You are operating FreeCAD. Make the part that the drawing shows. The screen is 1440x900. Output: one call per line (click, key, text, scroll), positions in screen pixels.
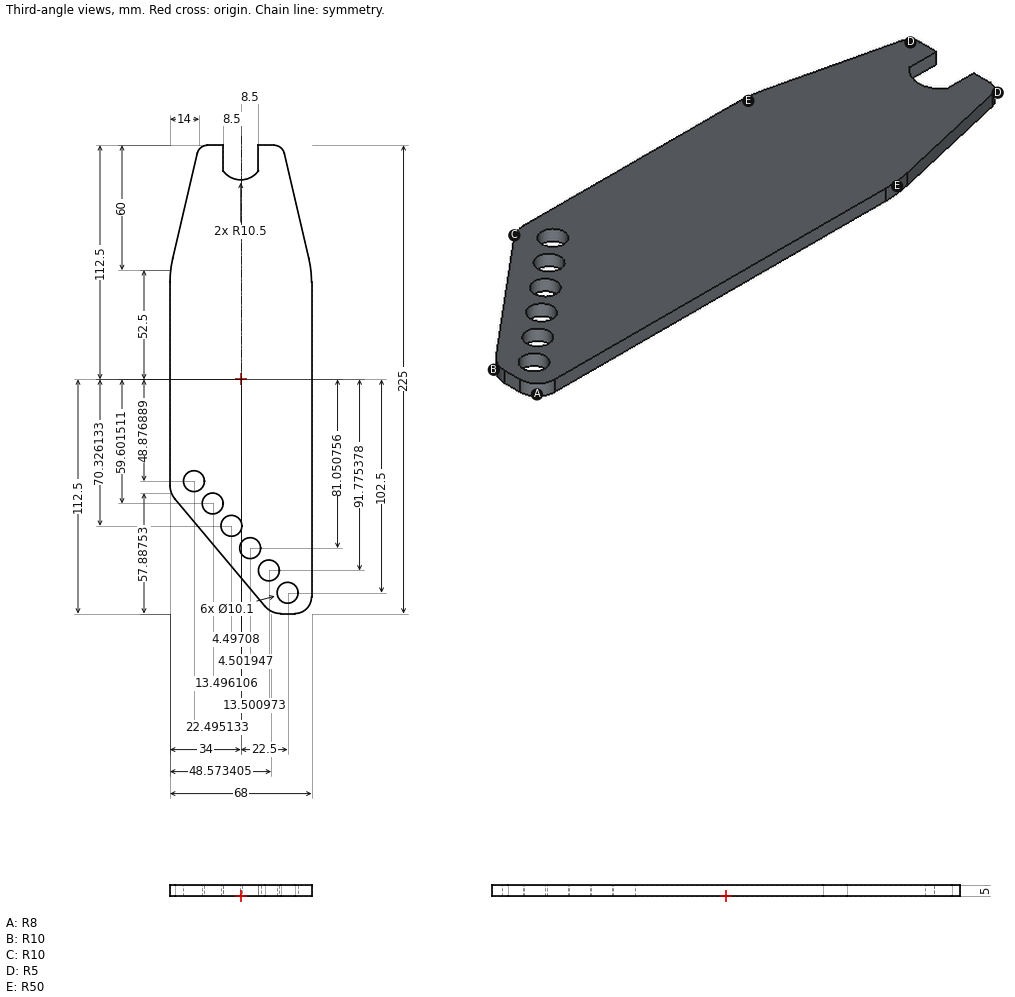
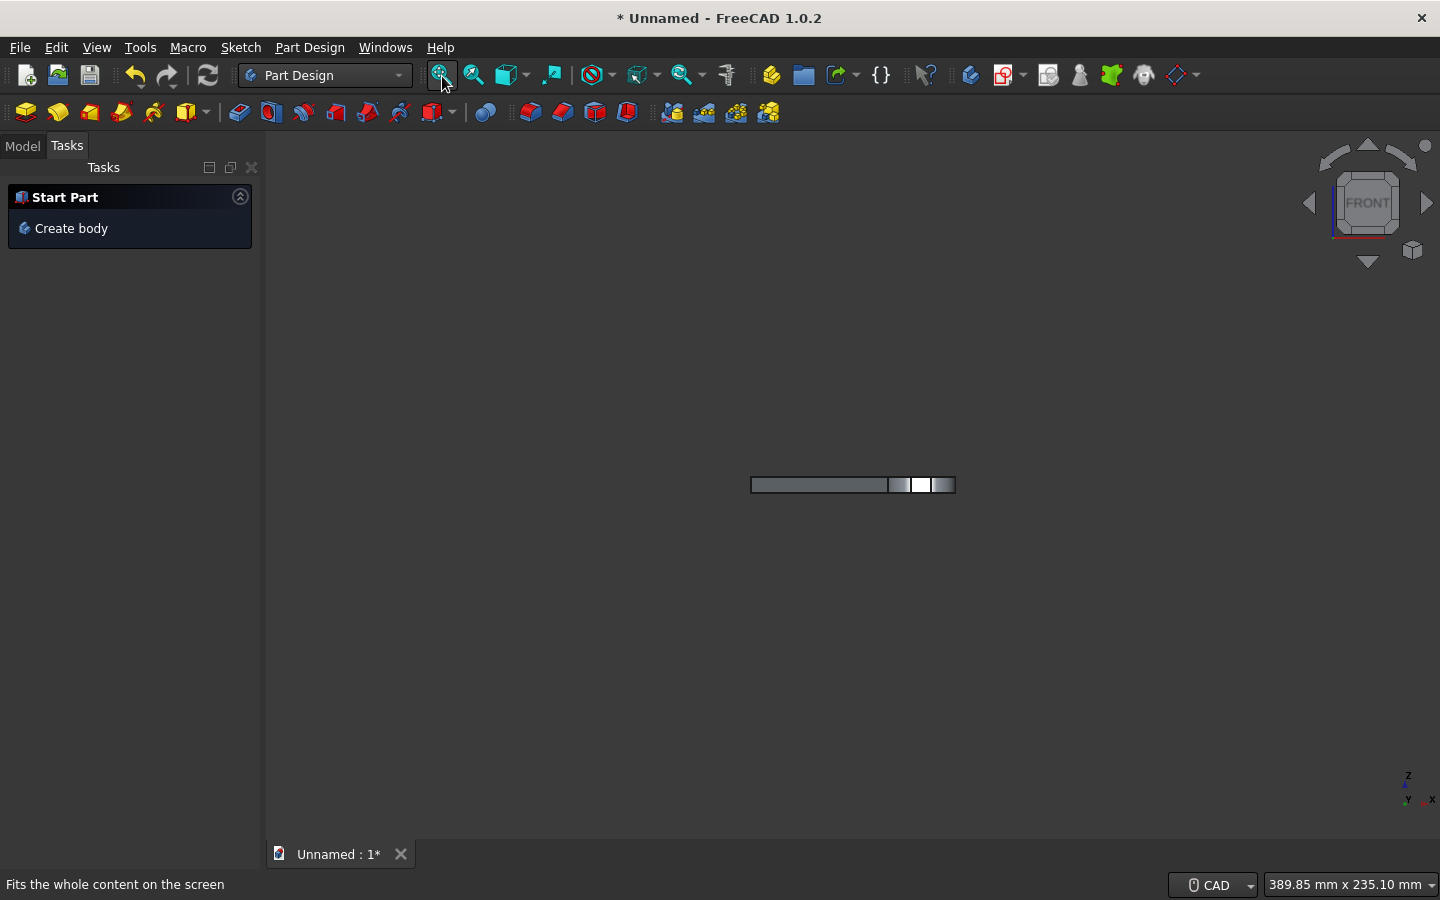
key(0)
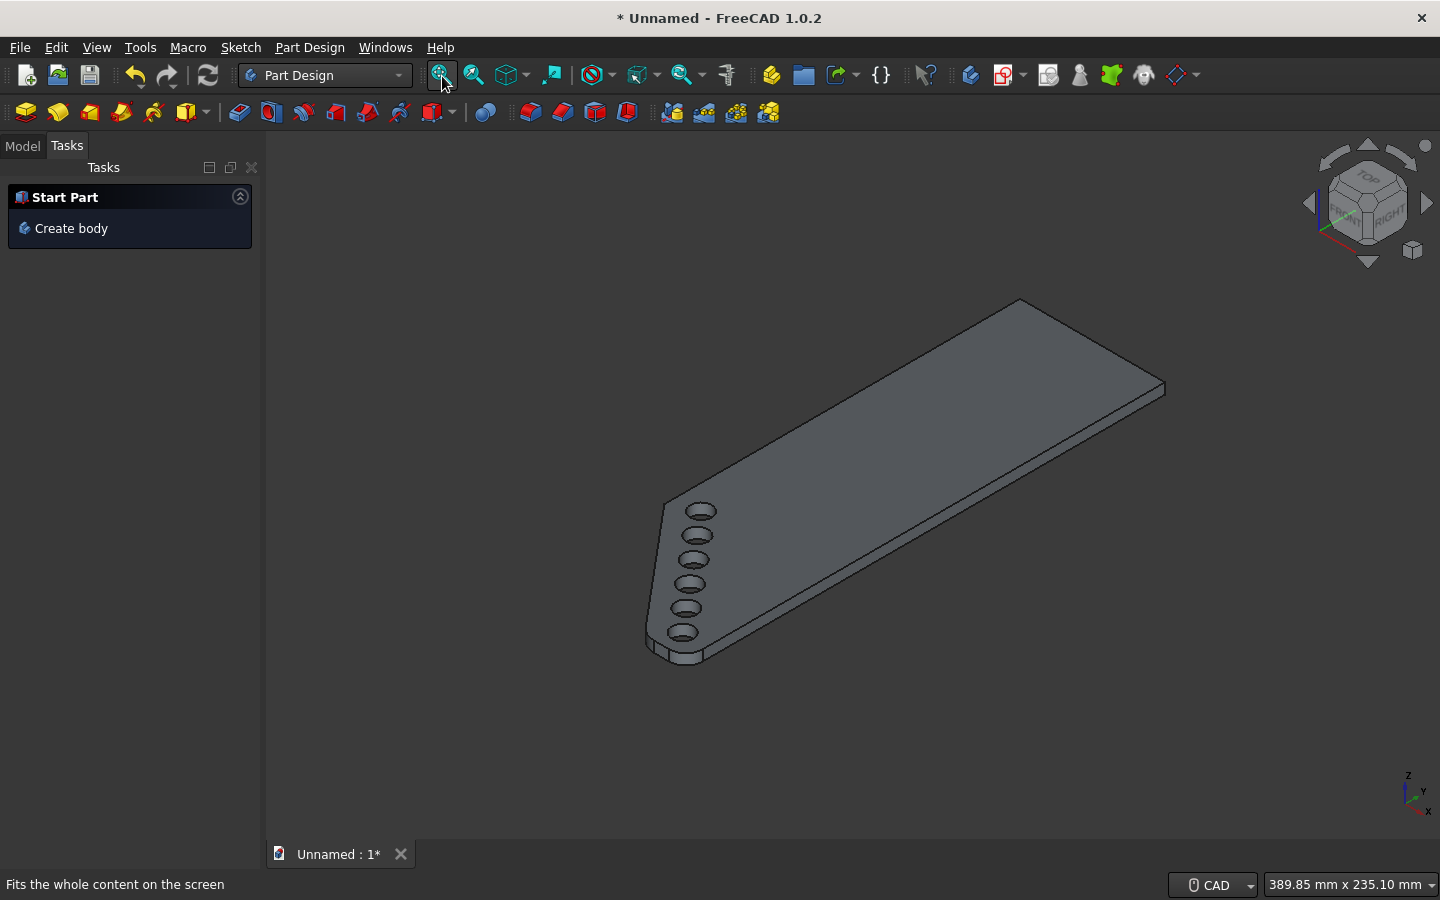
click(990, 399)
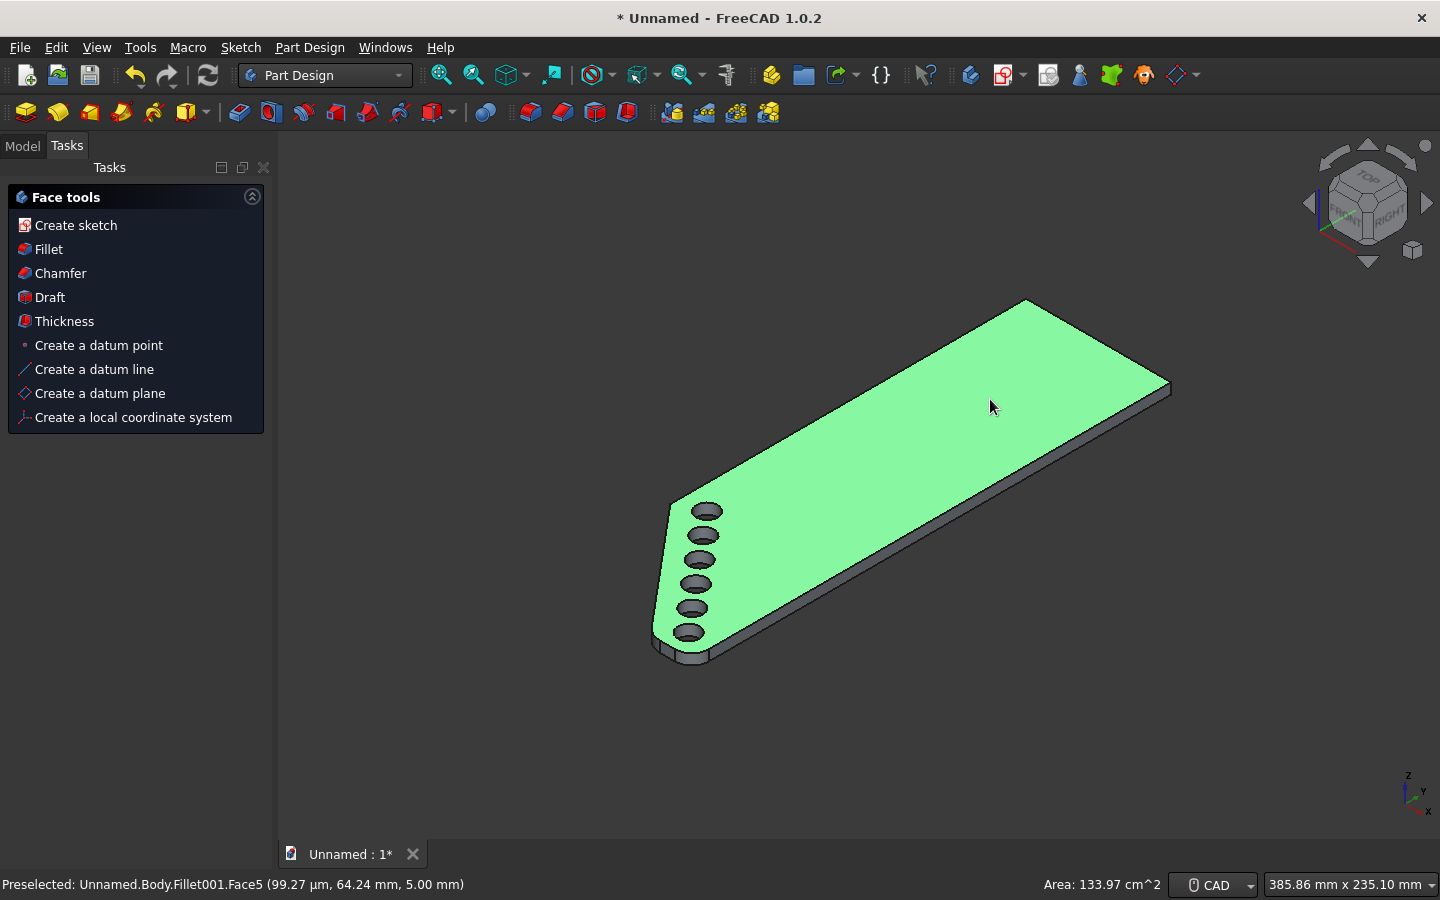
click(1004, 76)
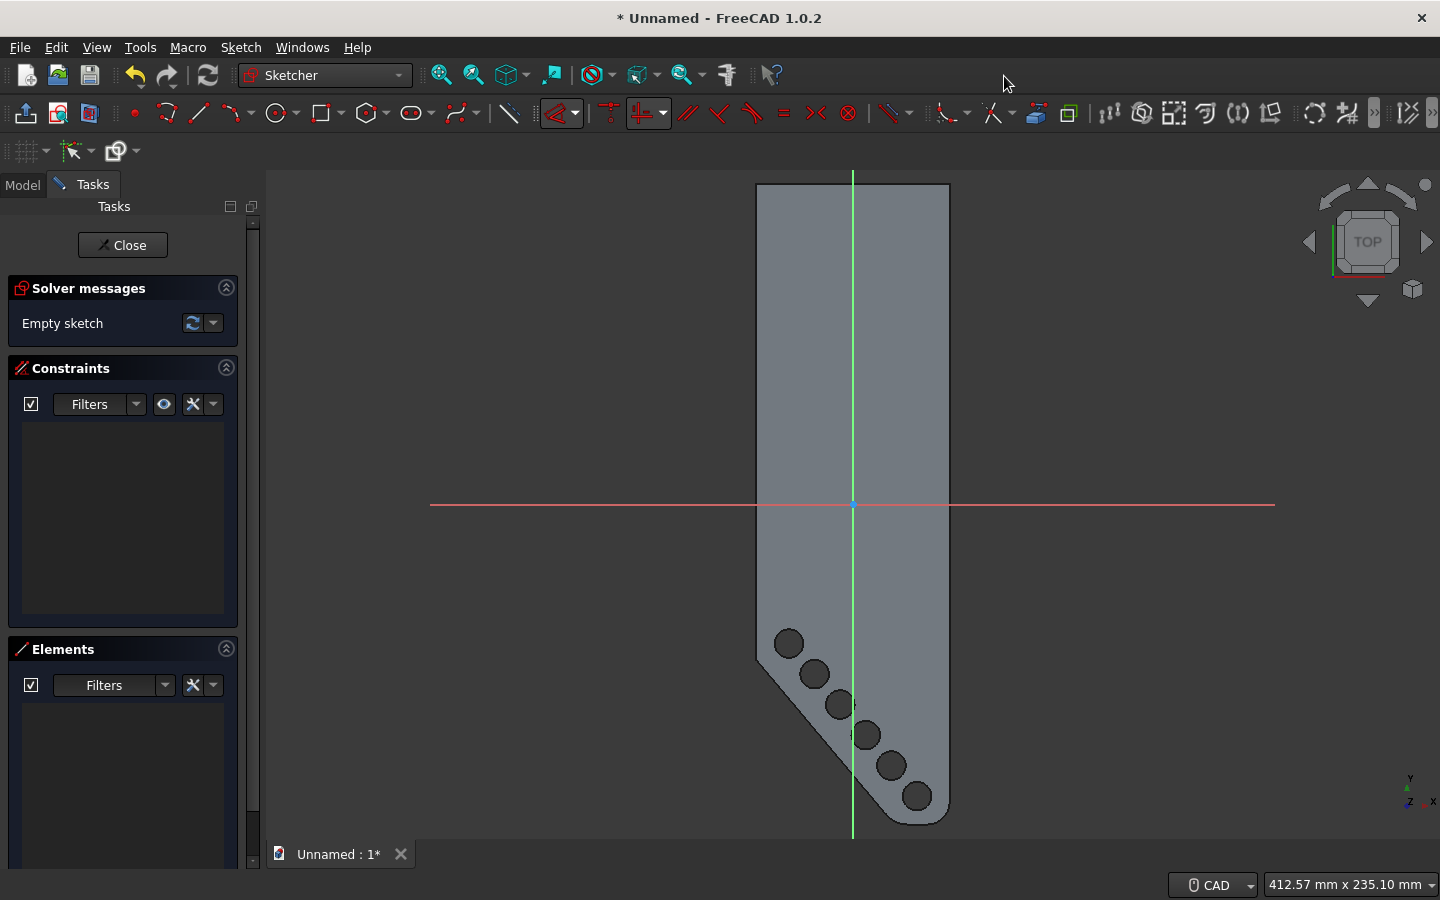
scroll(784, 504, down, 5)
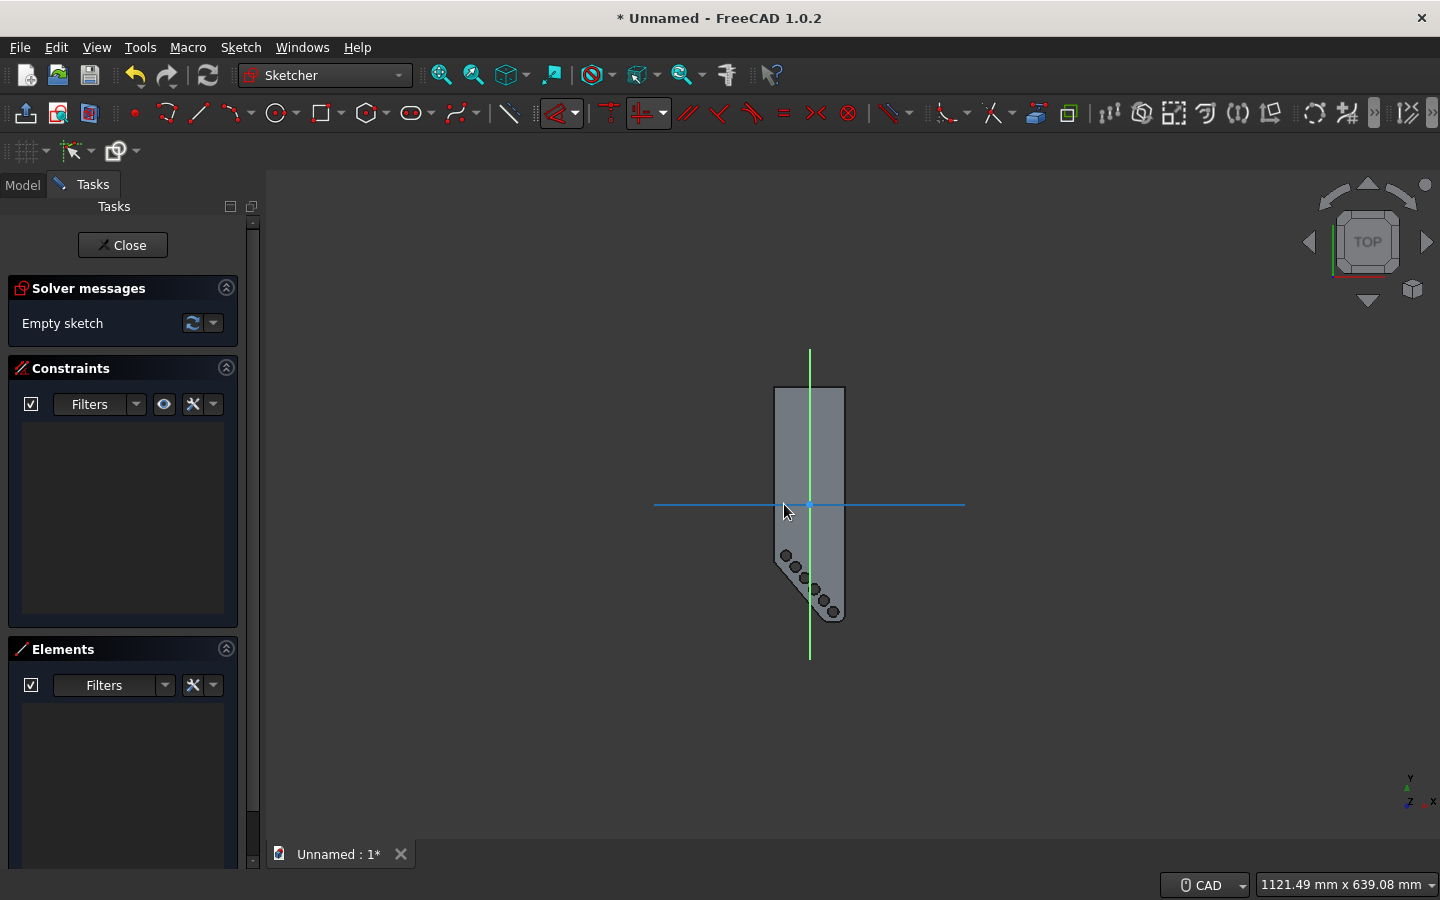
scroll(811, 387, up, 15)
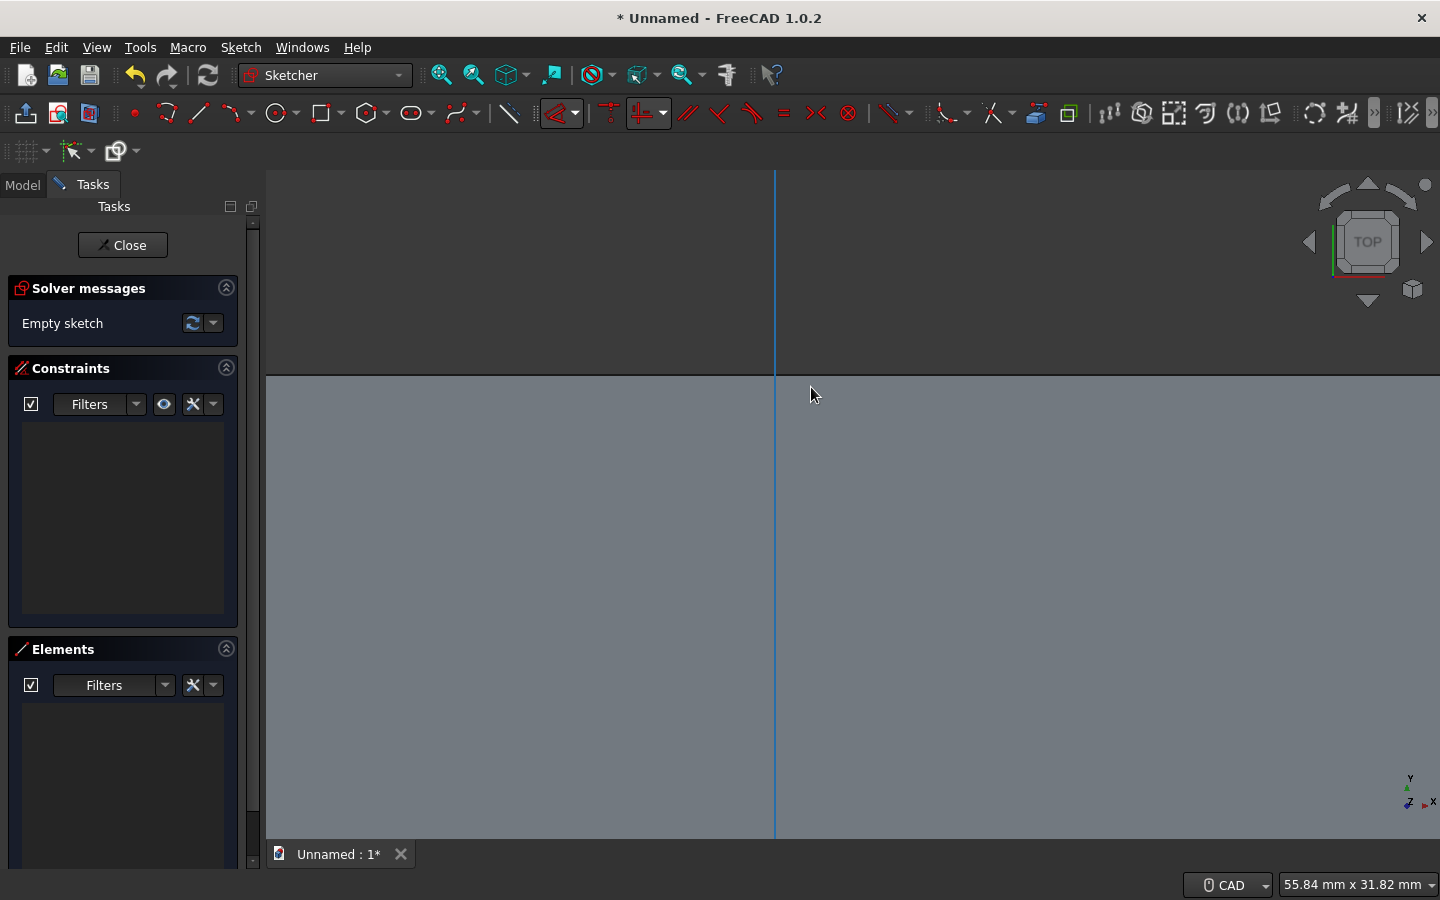
key(g)
key(l)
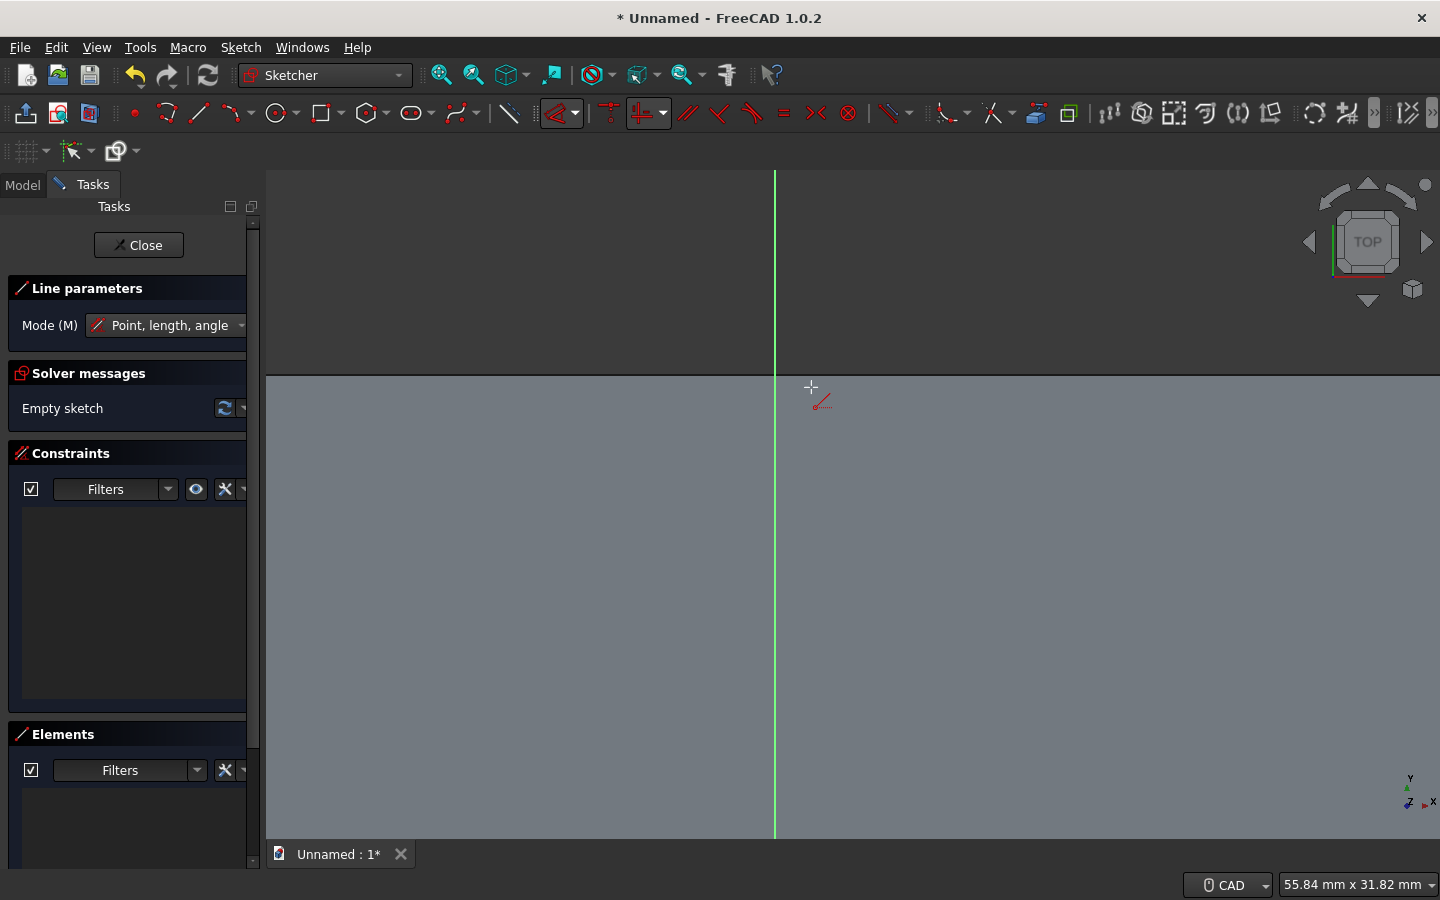
click(597, 375)
click(597, 635)